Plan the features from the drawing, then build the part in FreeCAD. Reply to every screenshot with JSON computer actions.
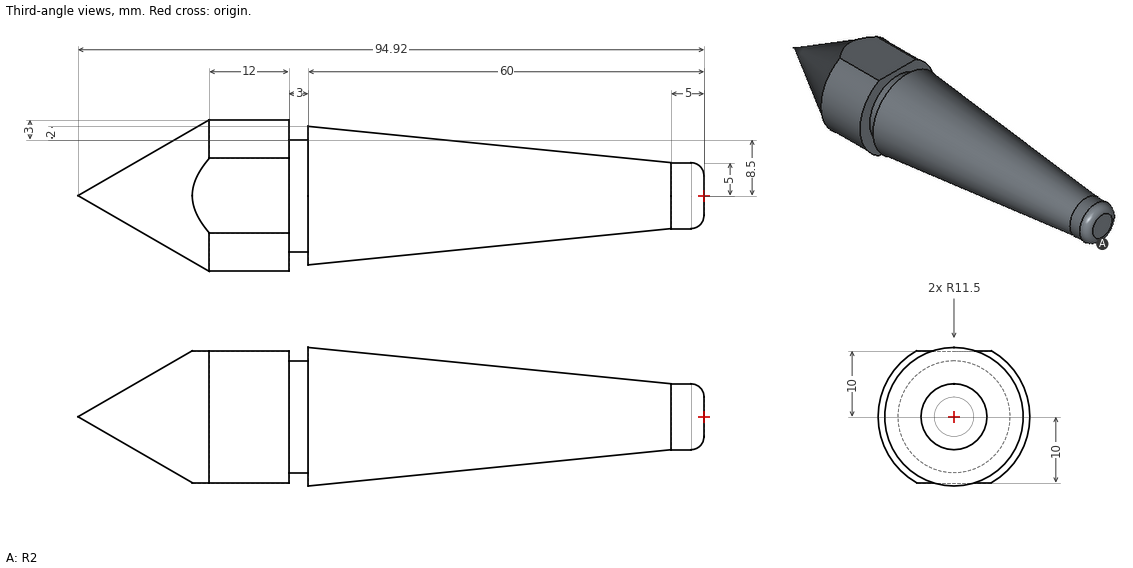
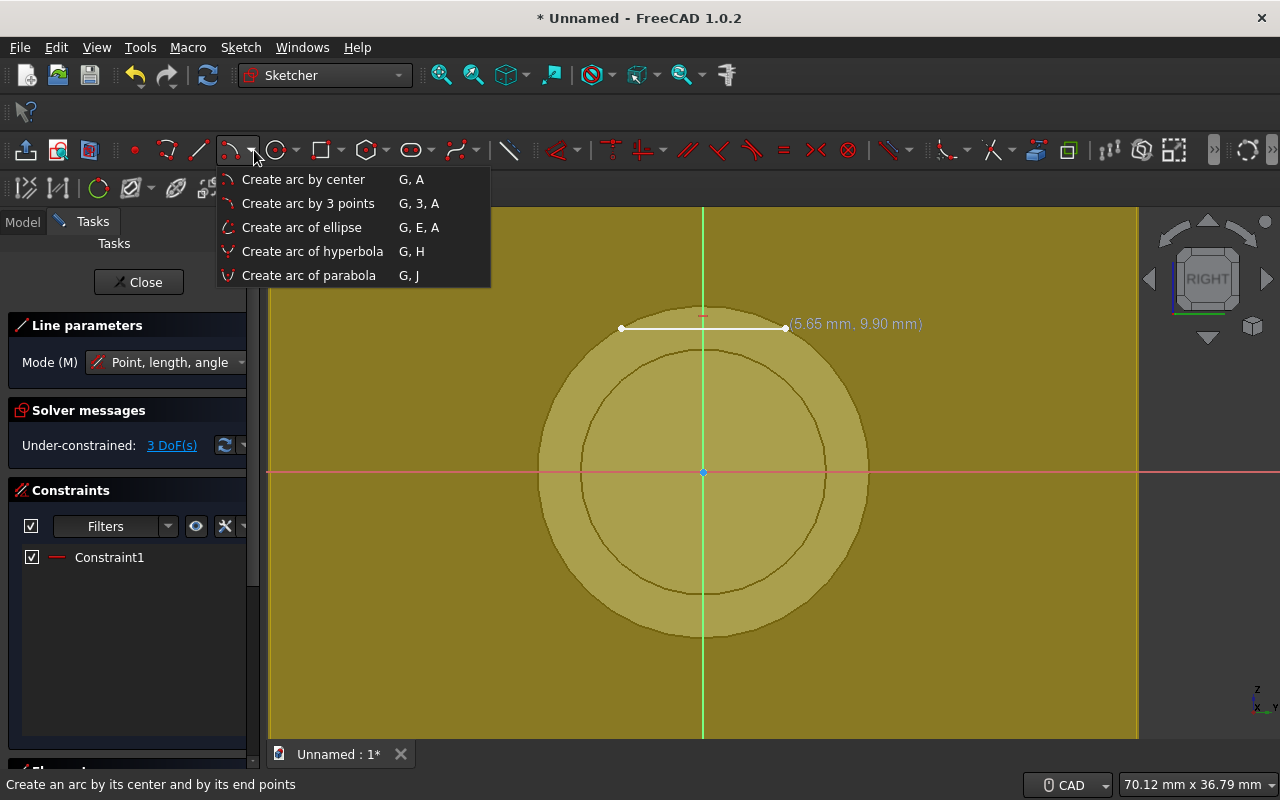
{"action": "left_click", "coordinate": [354, 203]}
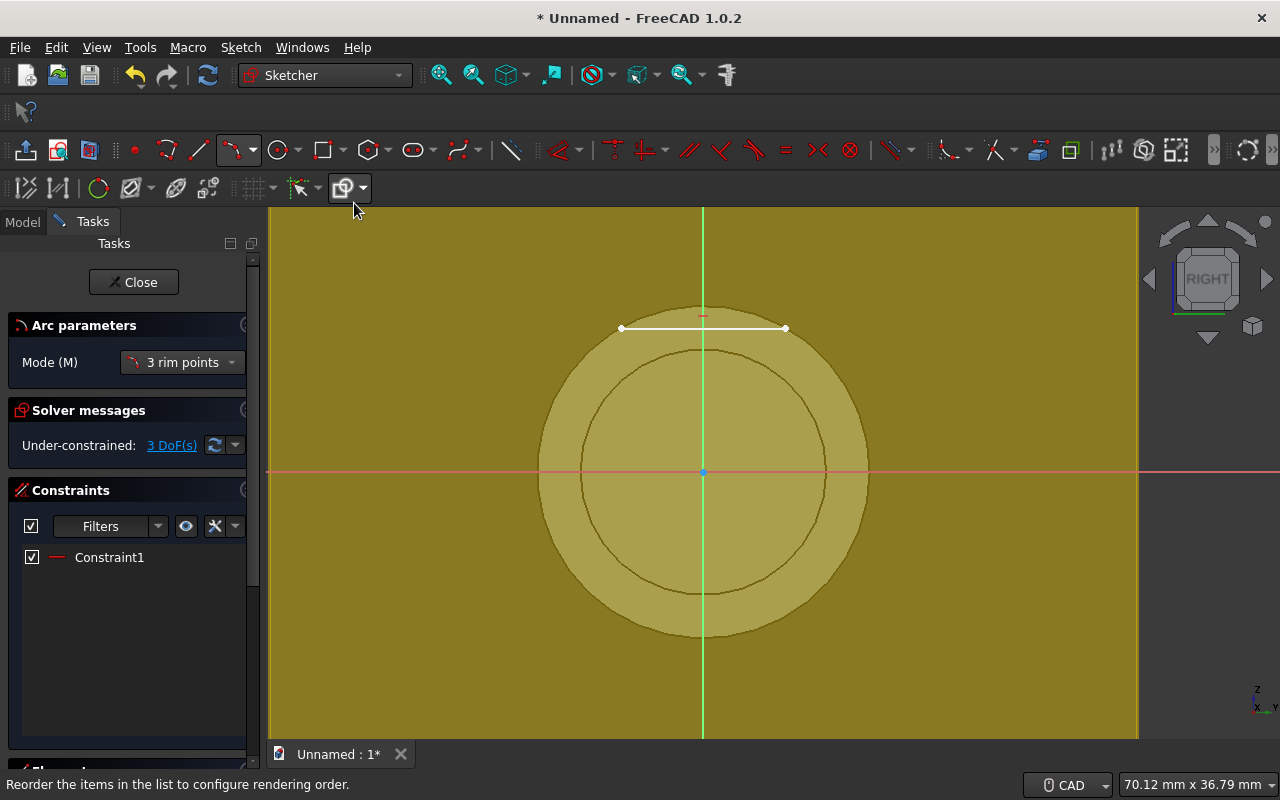
{"action": "left_click", "coordinate": [785, 329]}
{"action": "left_click", "coordinate": [621, 329]}
{"action": "left_click", "coordinate": [720, 307]}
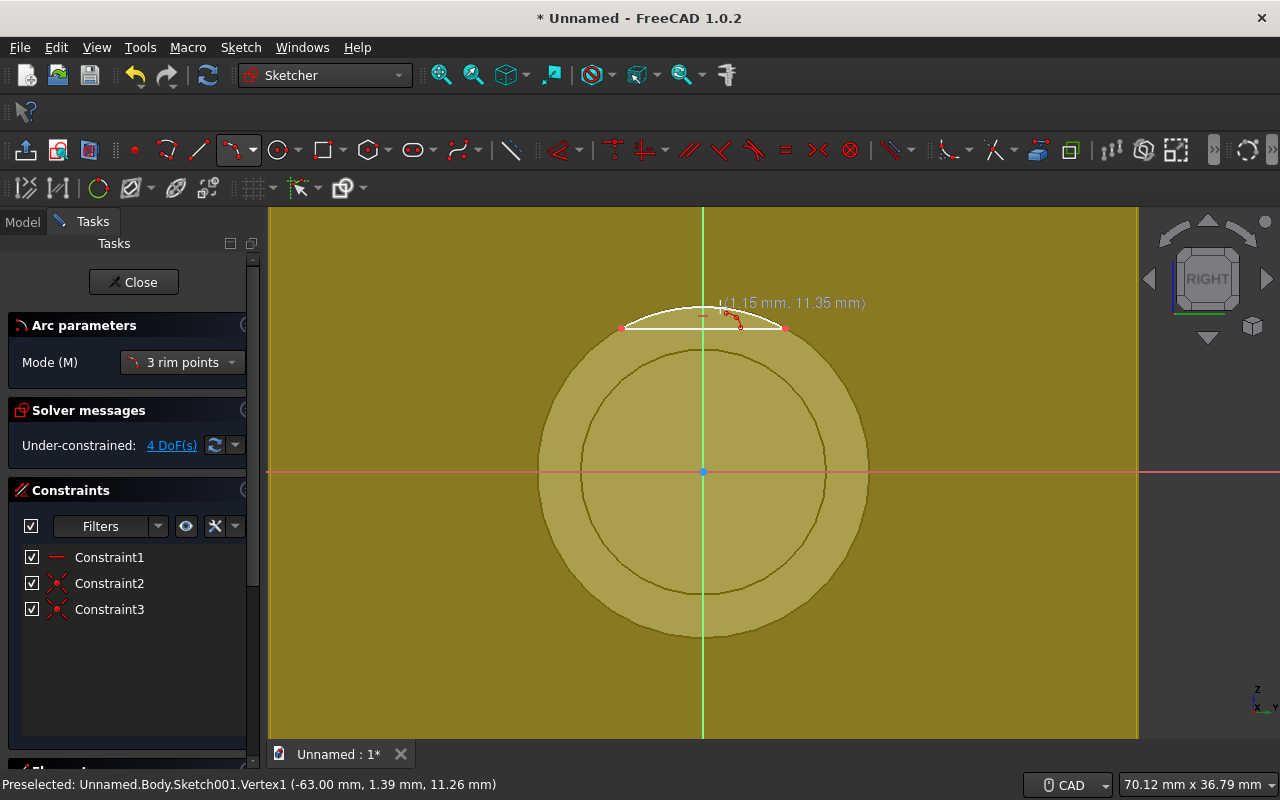
{"action": "left_click", "coordinate": [200, 150]}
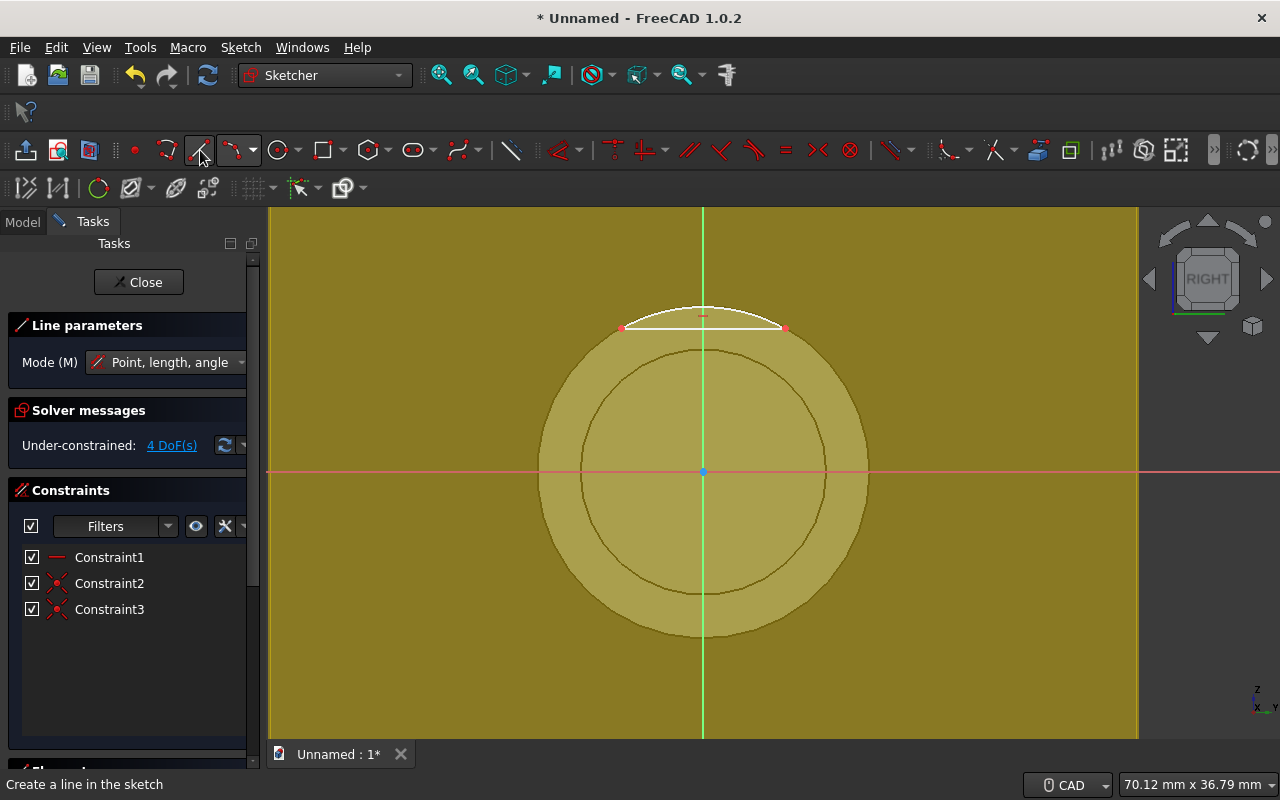
{"action": "left_click", "coordinate": [785, 617]}
{"action": "left_click", "coordinate": [621, 617]}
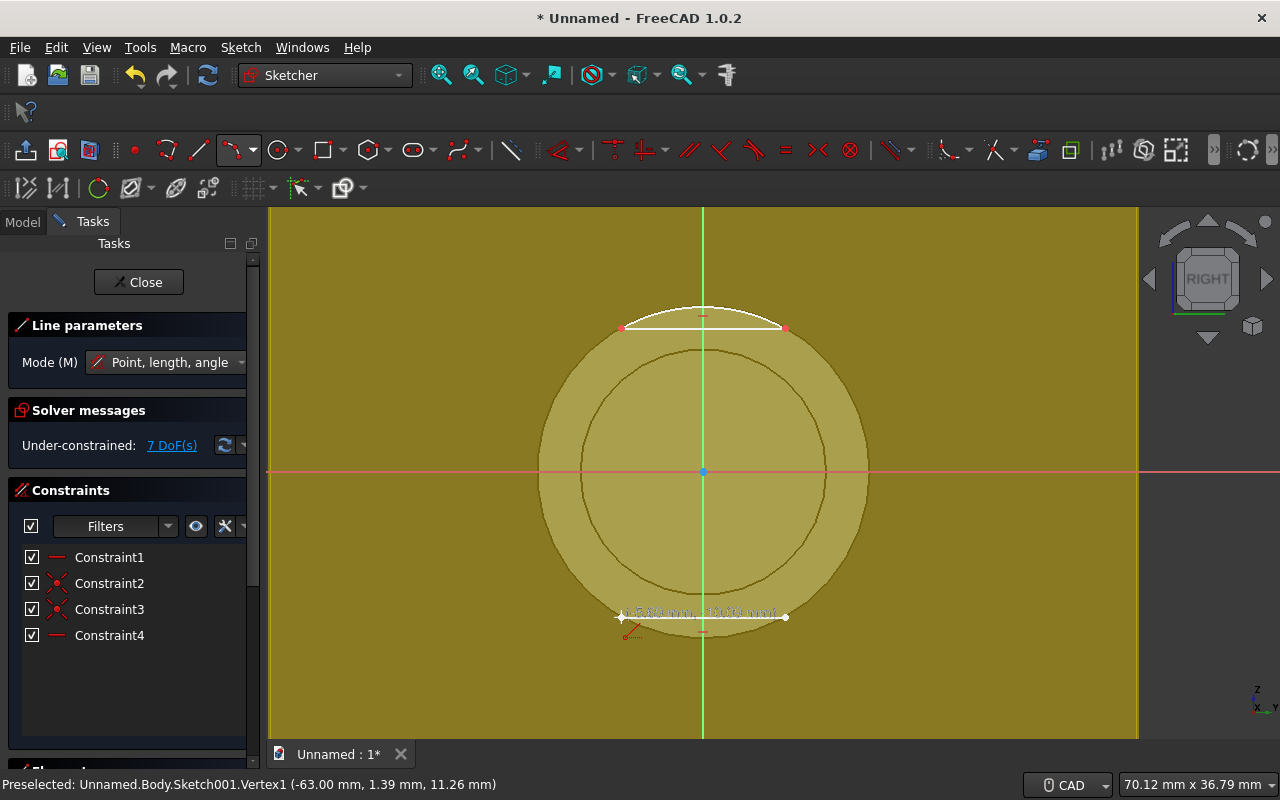
{"action": "left_click", "coordinate": [232, 150]}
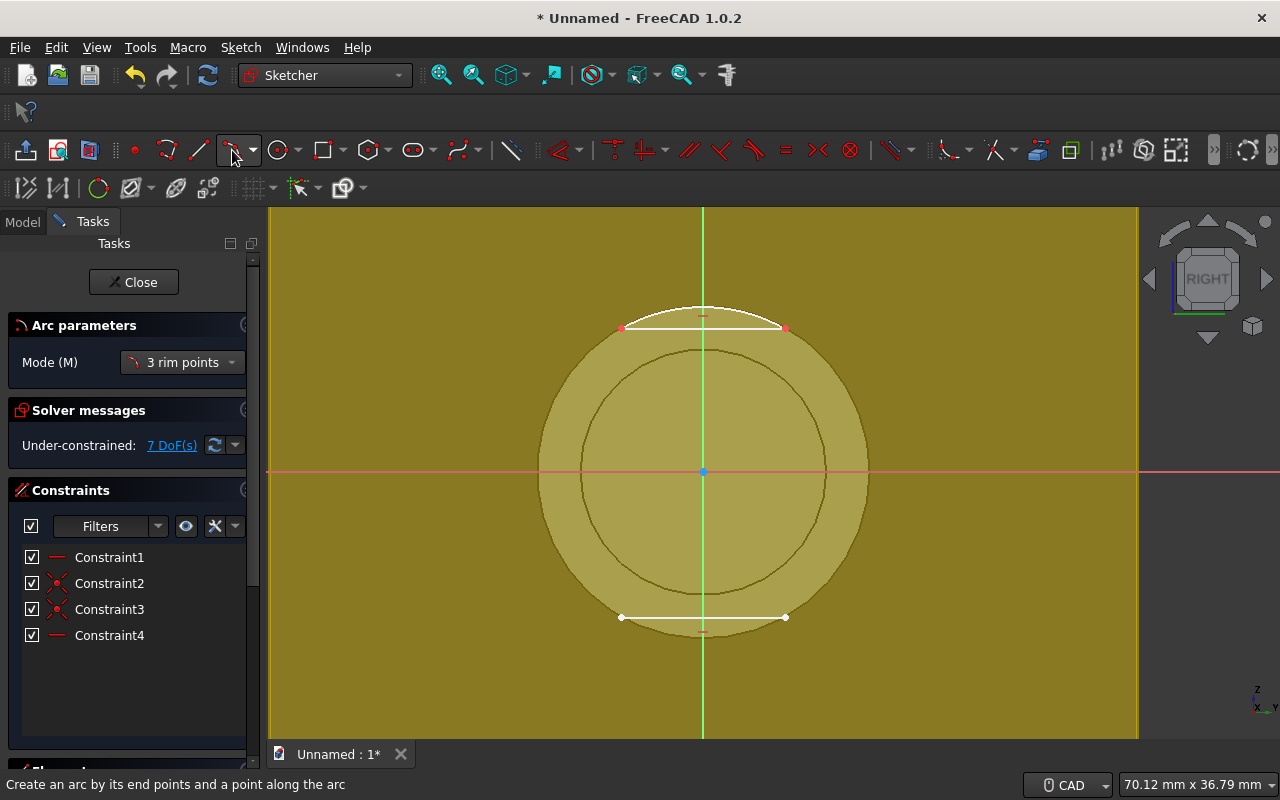
{"action": "left_click", "coordinate": [621, 618]}
{"action": "left_click", "coordinate": [785, 618]}
{"action": "left_click", "coordinate": [686, 638]}
{"action": "key", "text": "Escape"}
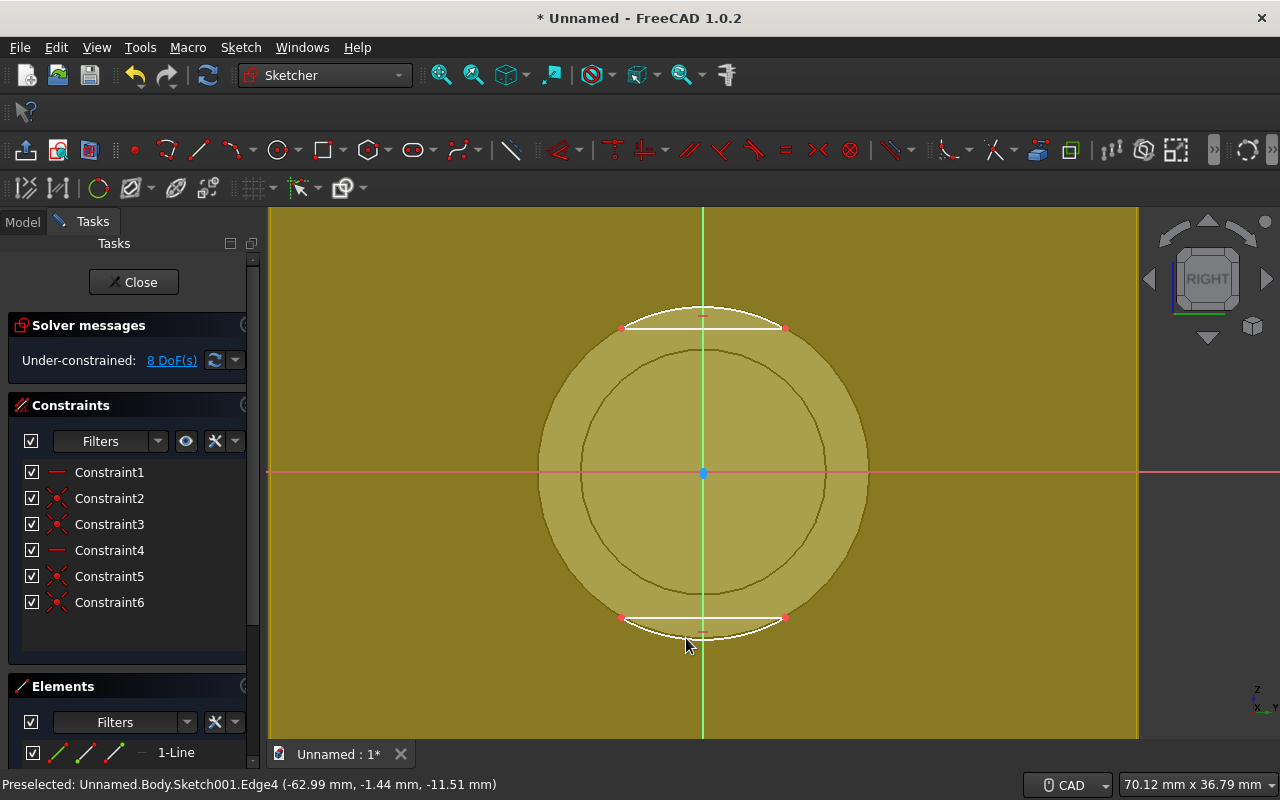
{"action": "left_click", "coordinate": [737, 311]}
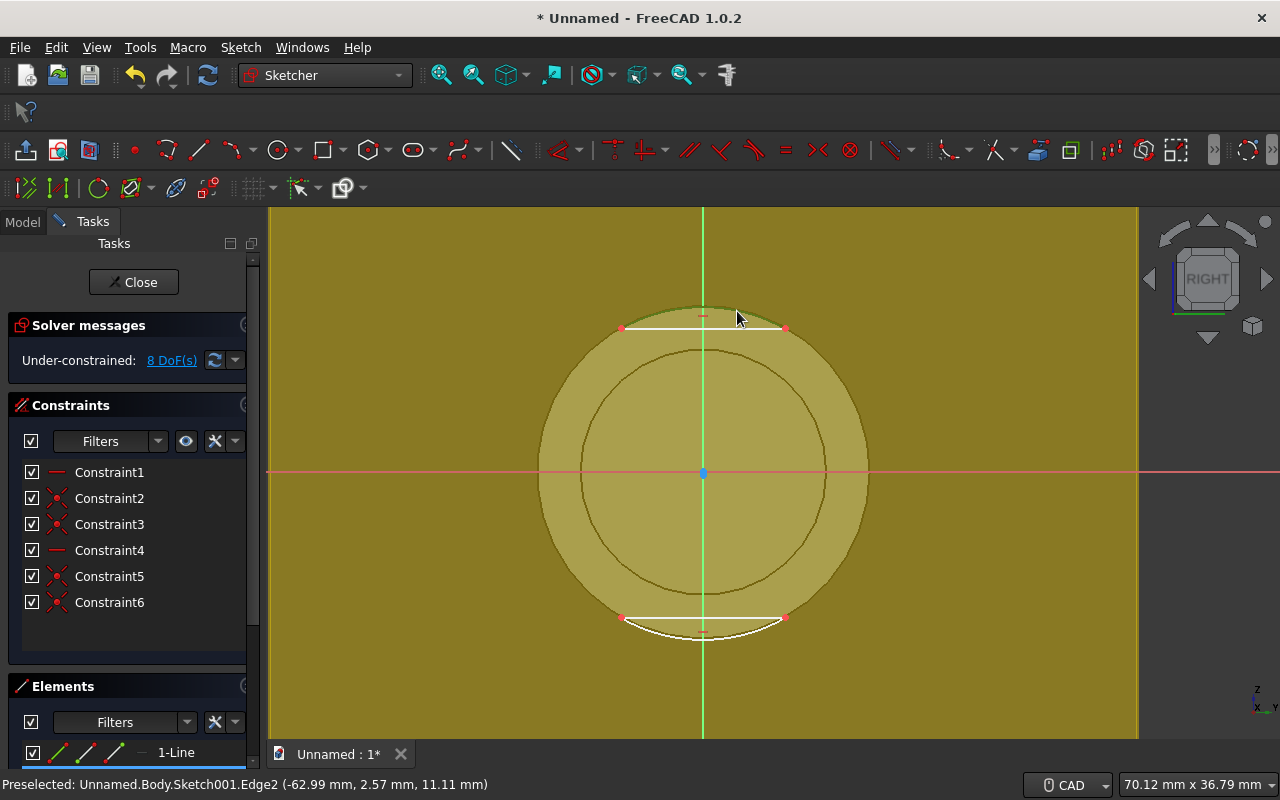
{"action": "left_click", "coordinate": [669, 636]}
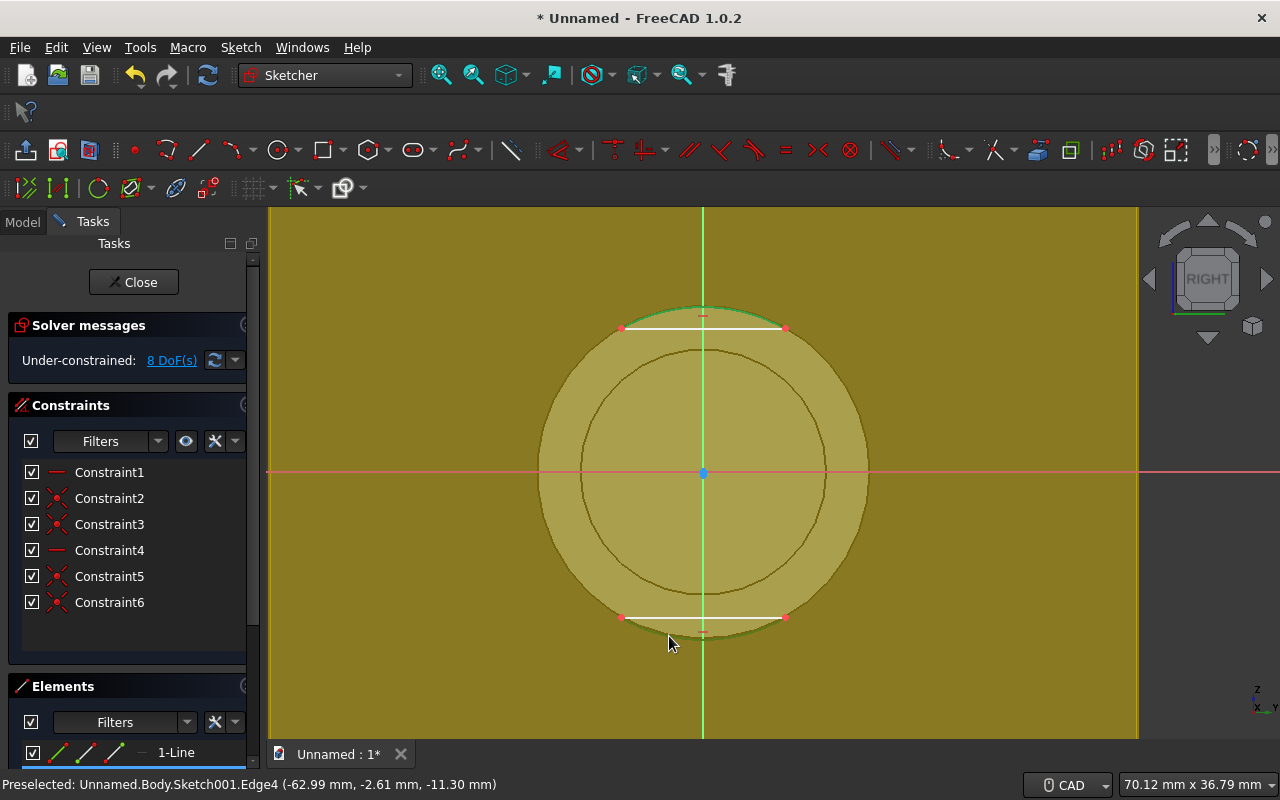
{"action": "key", "text": "c"}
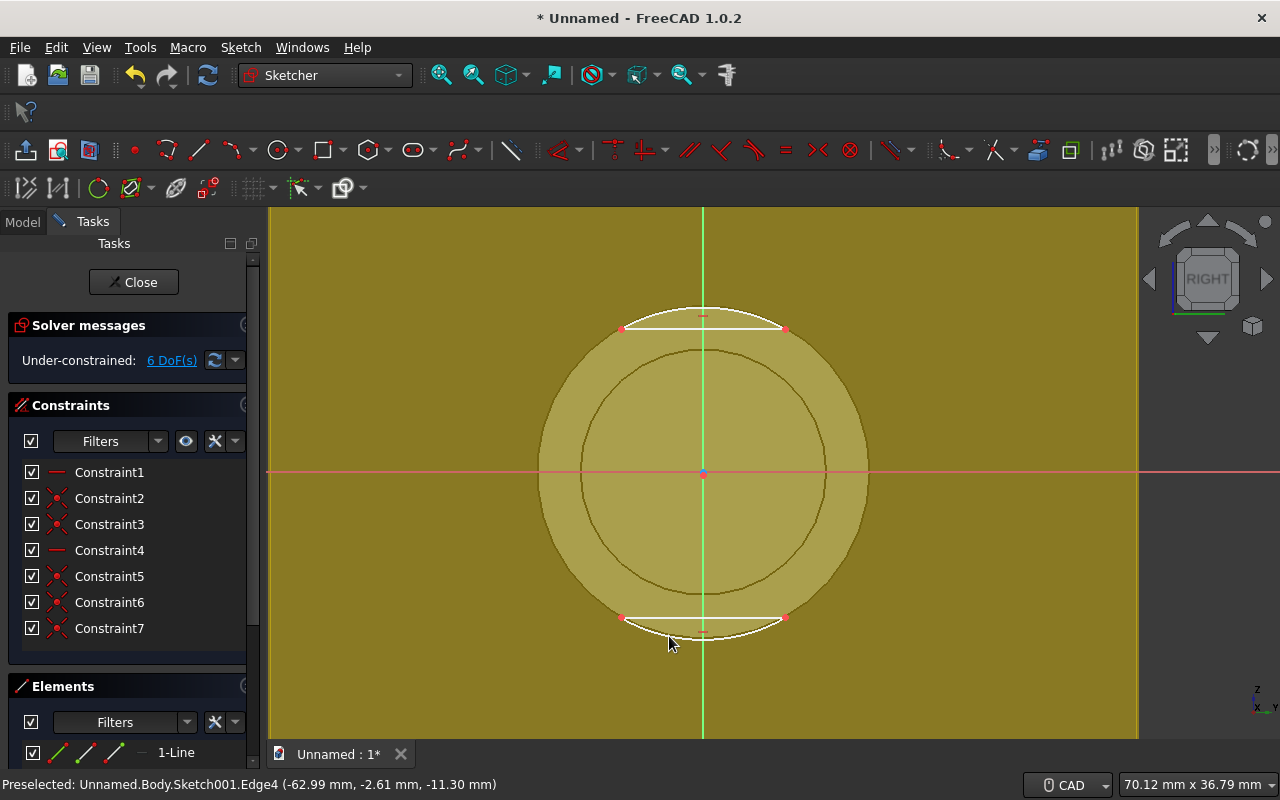
{"action": "left_click_drag", "start_coordinate": [693, 462], "coordinate": [713, 485]}